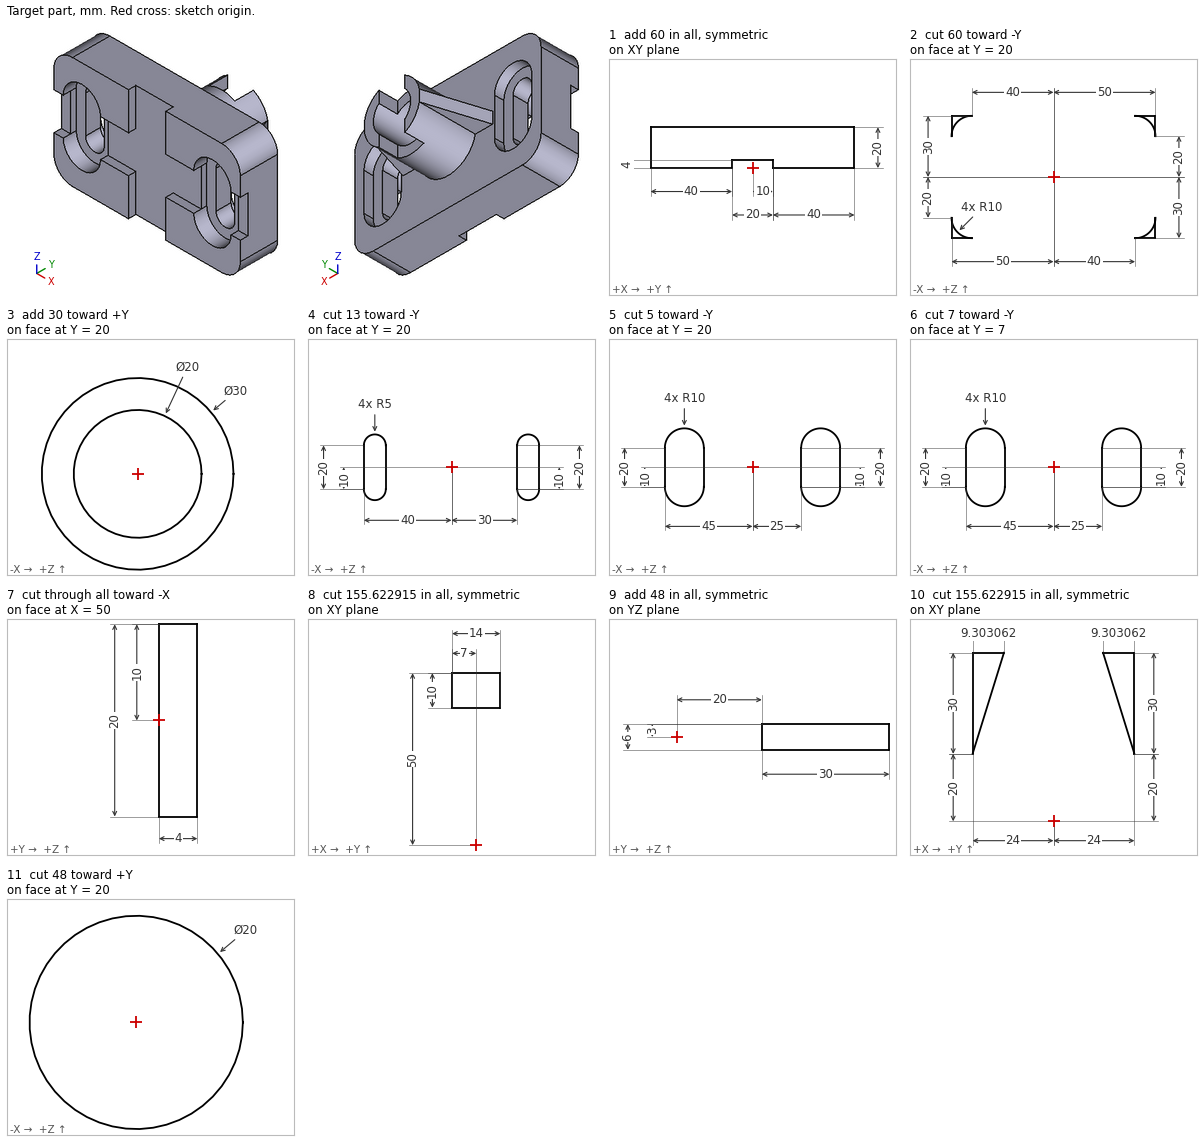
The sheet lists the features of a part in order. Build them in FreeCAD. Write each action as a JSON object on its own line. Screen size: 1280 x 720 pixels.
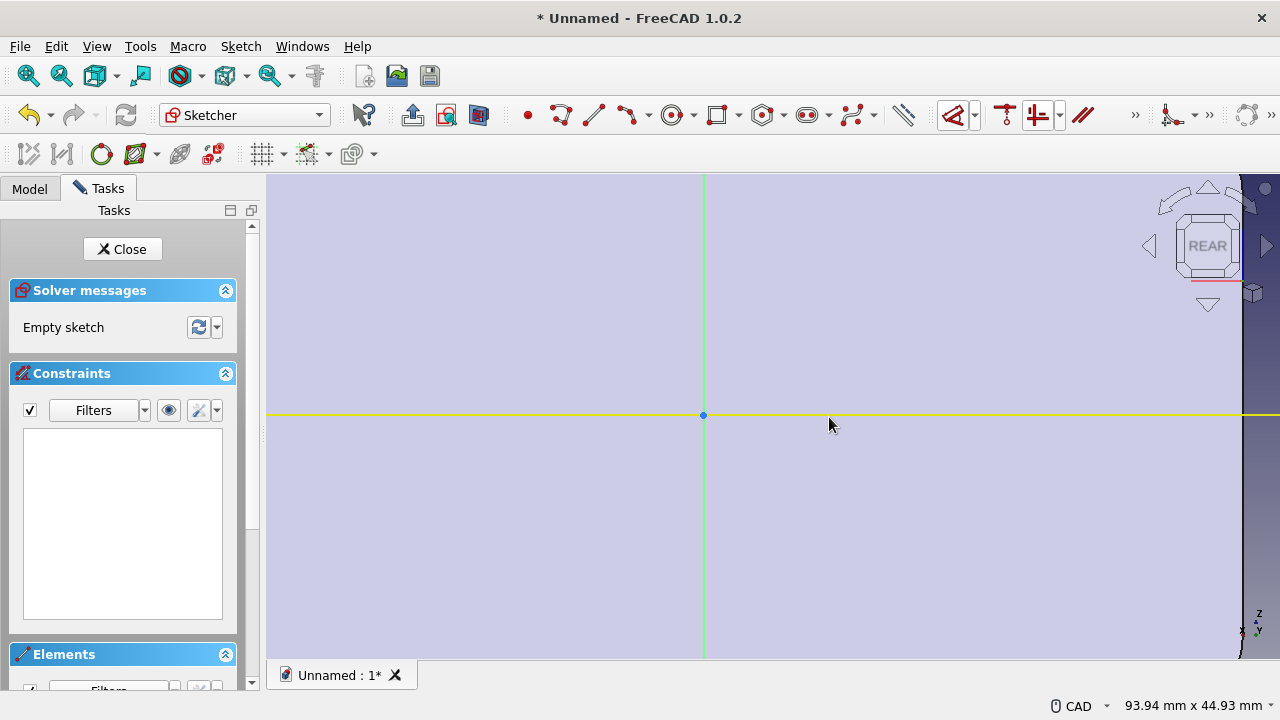
{"action": "key", "text": "g c"}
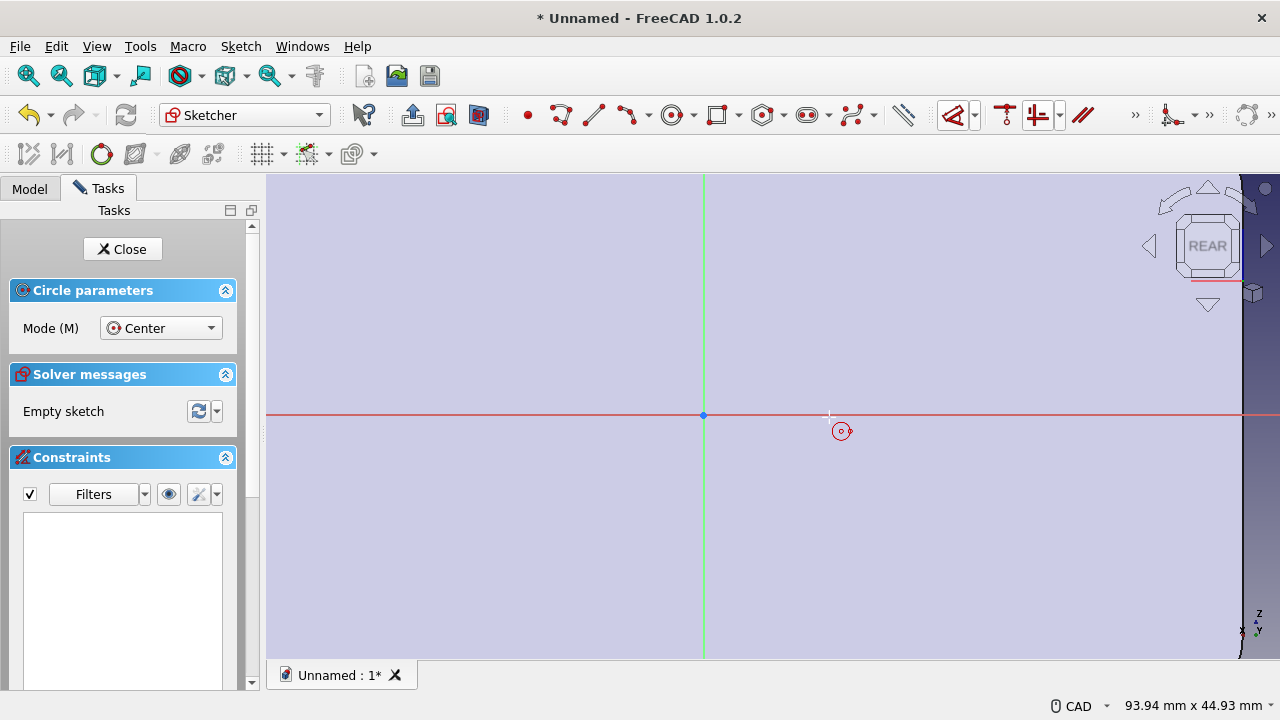
{"action": "left_click", "coordinate": [704, 415]}
{"action": "left_click", "coordinate": [818, 301]}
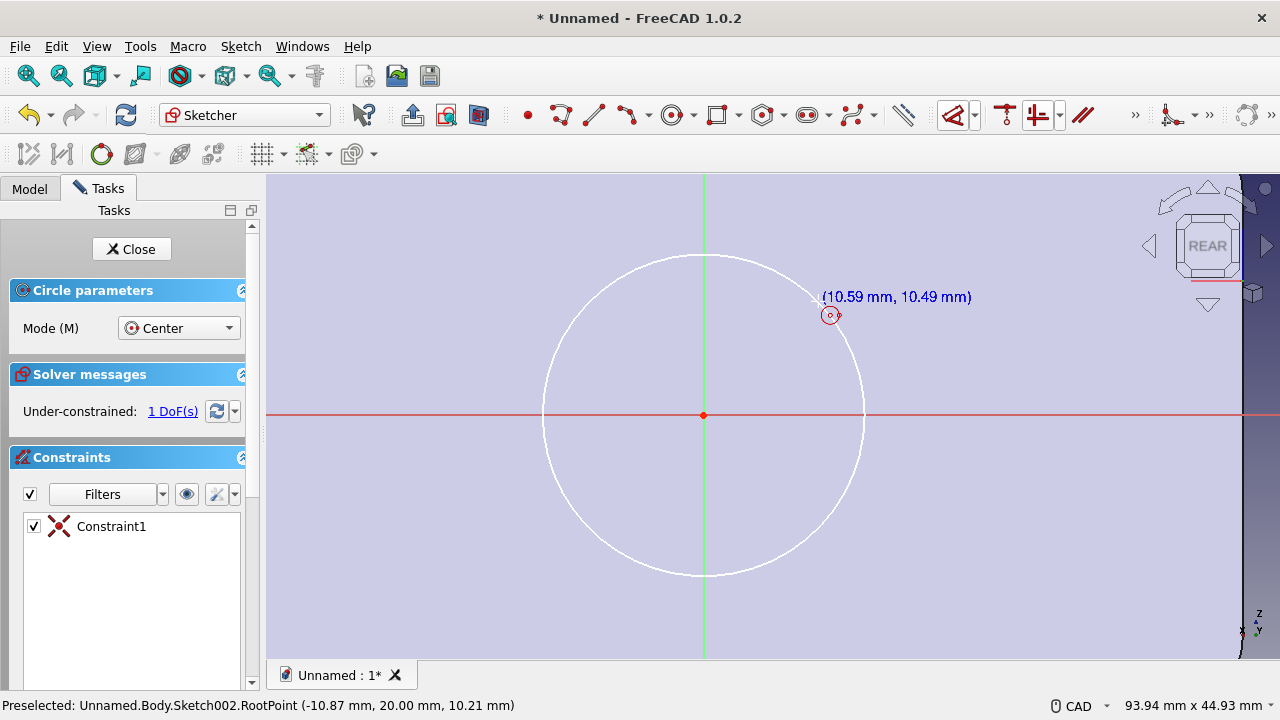
{"action": "left_click", "coordinate": [704, 415]}
{"action": "left_click", "coordinate": [780, 339]}
{"action": "key", "text": "Escape"}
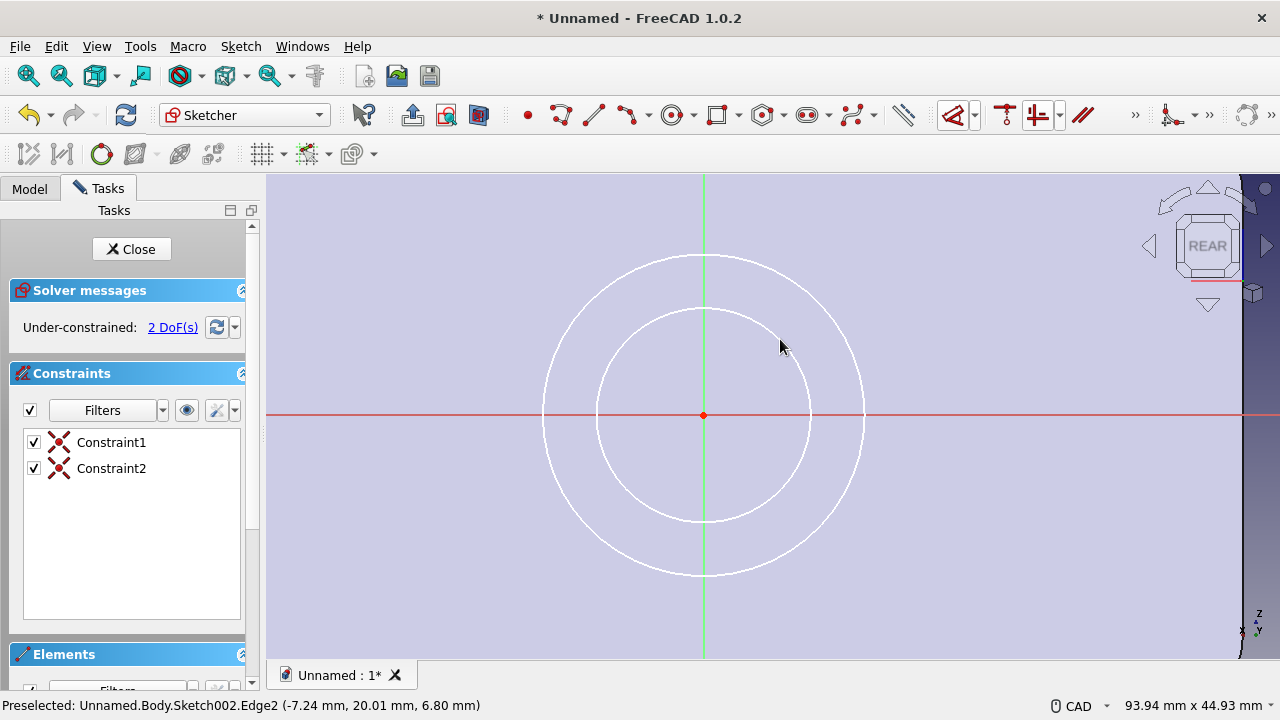
{"action": "left_click", "coordinate": [817, 301]}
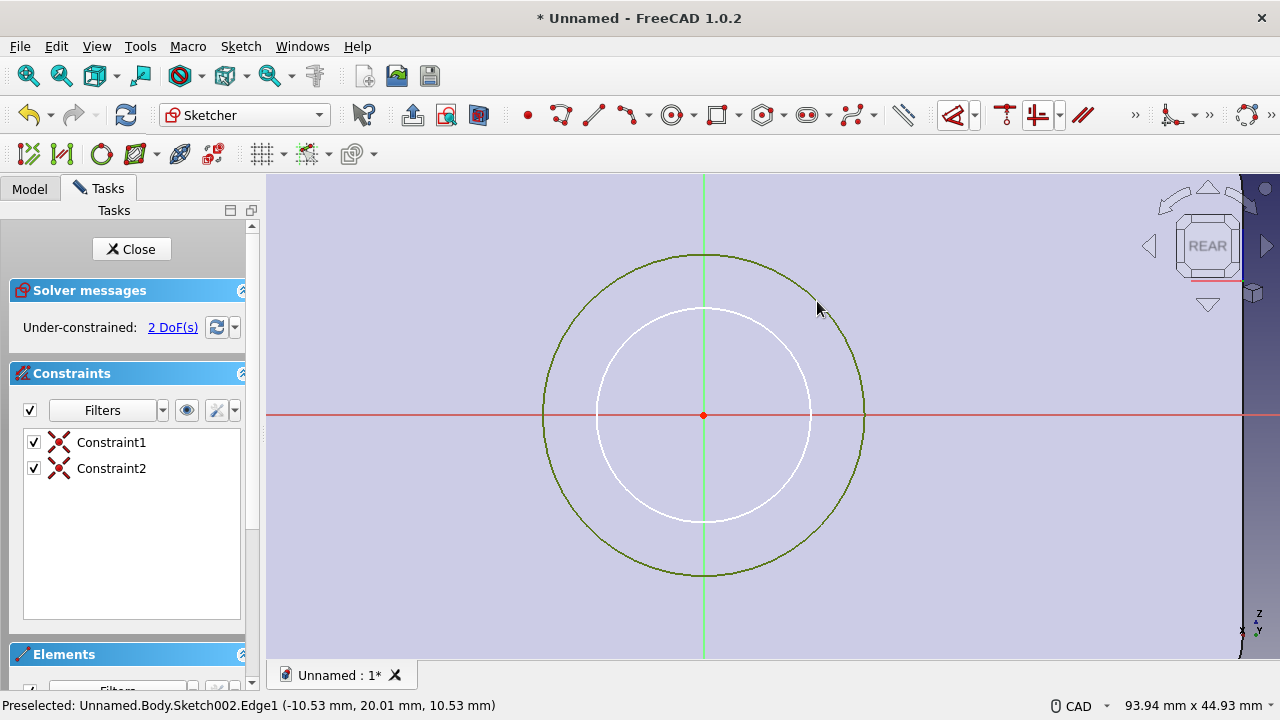
{"action": "key", "text": "k o"}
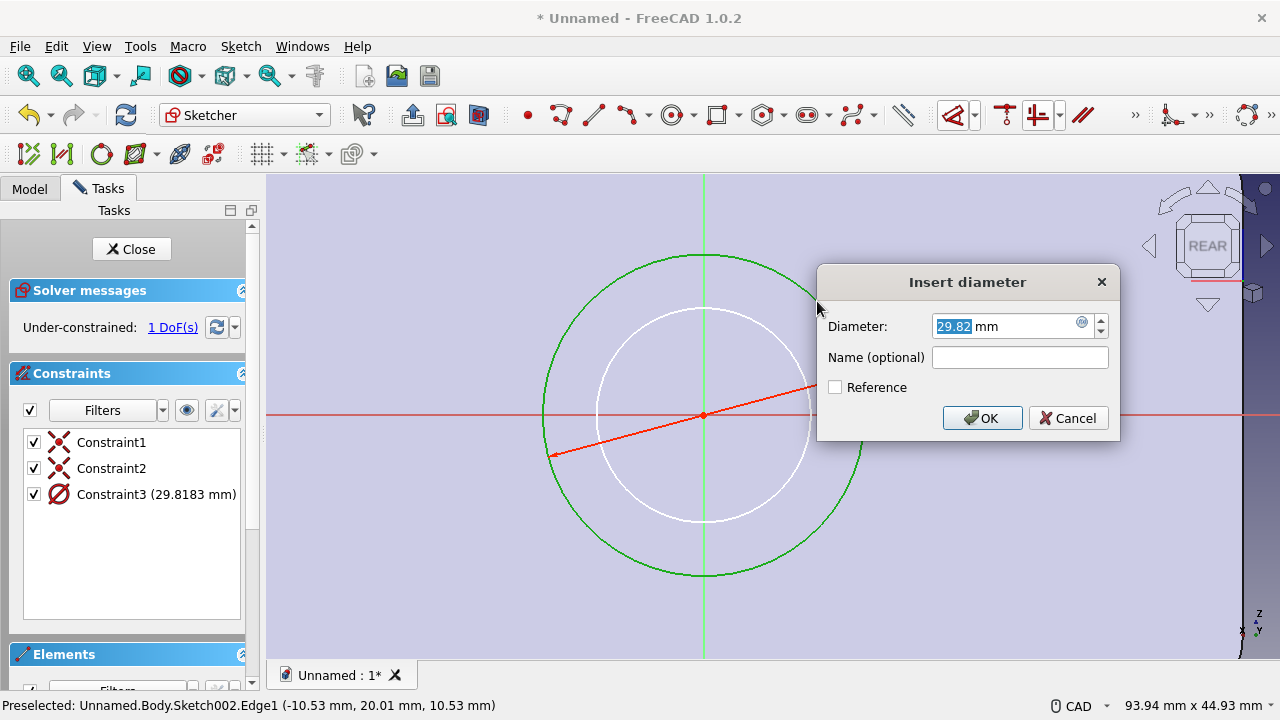
{"action": "type", "text": "30"}
{"action": "key", "text": "Return"}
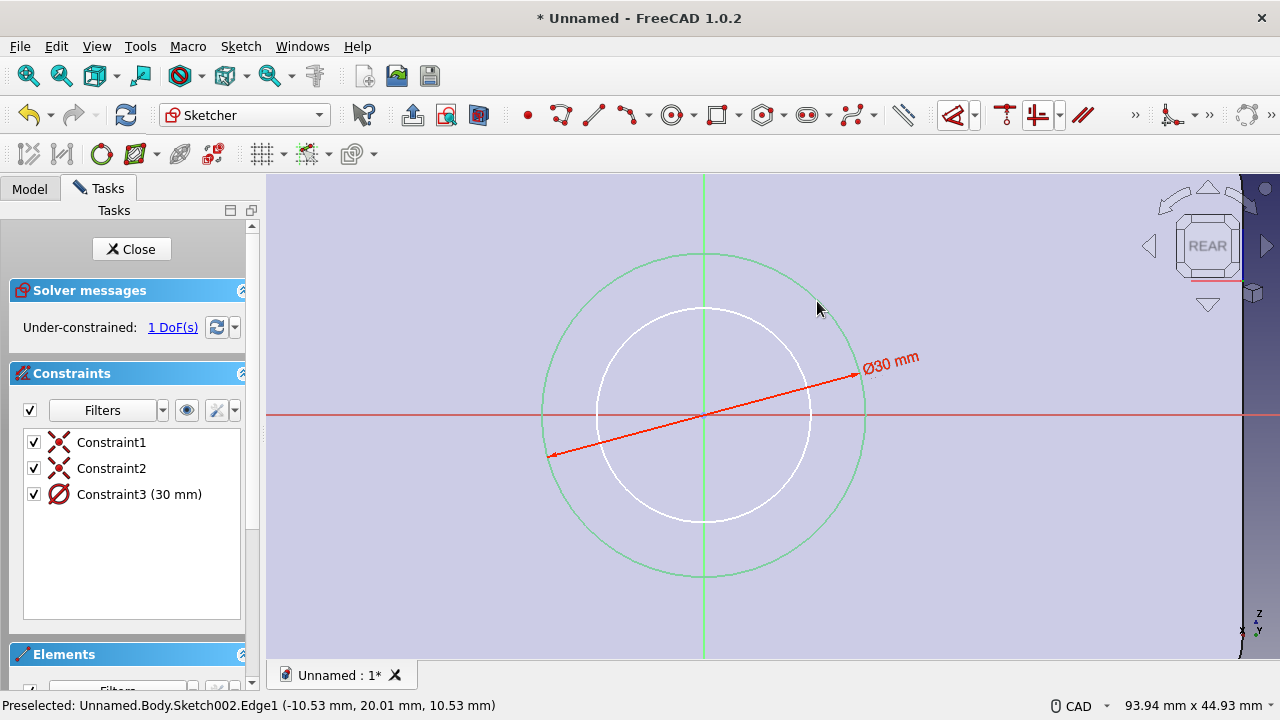
{"action": "left_click", "coordinate": [779, 339]}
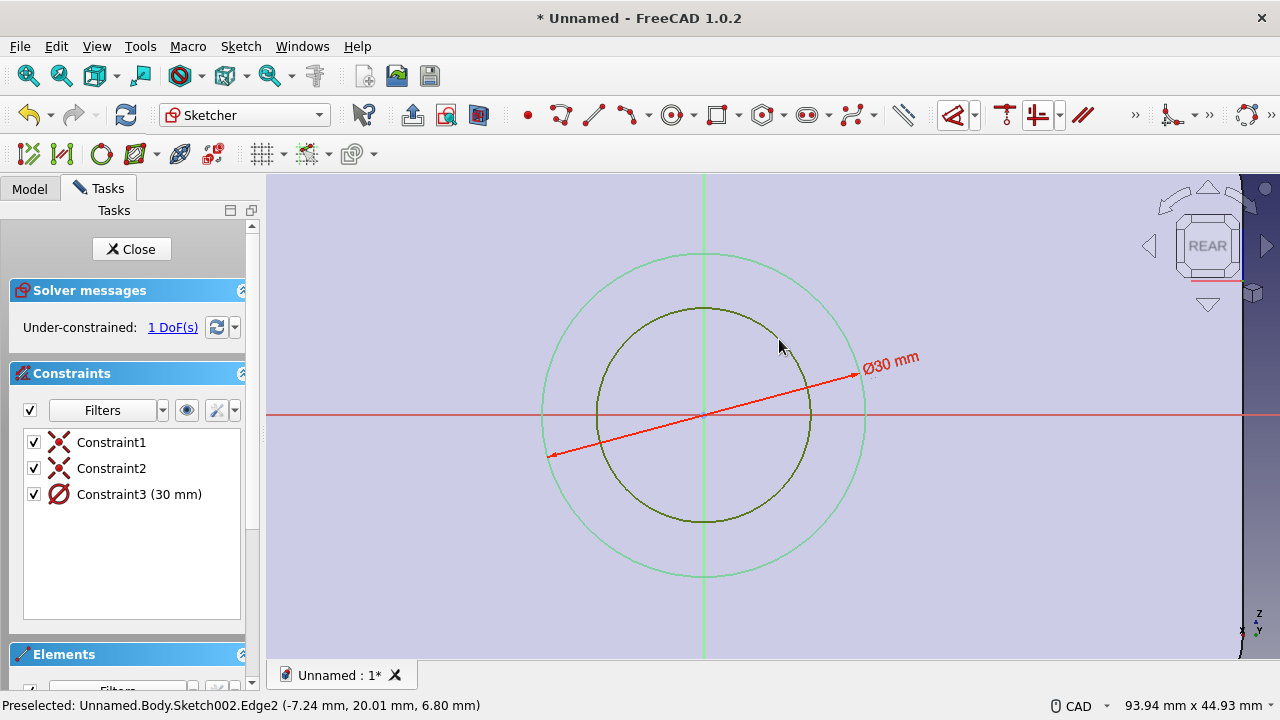
{"action": "key", "text": "k o"}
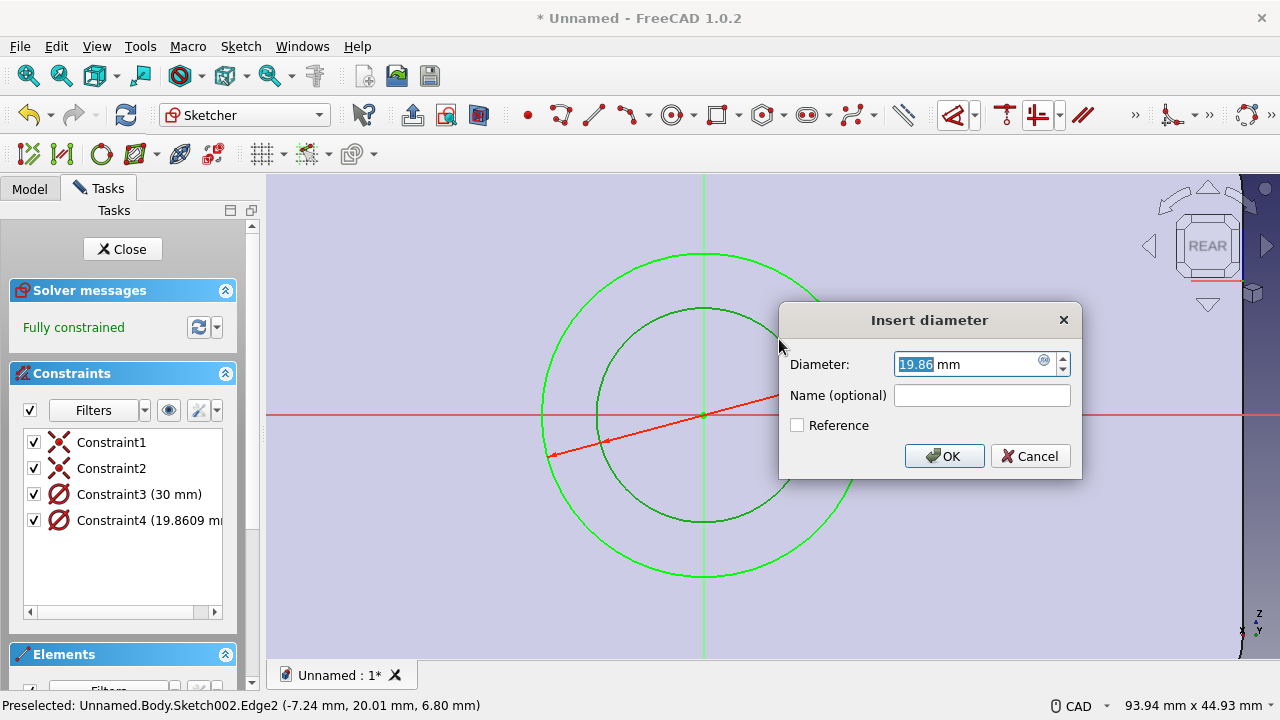
{"action": "type", "text": "20"}
{"action": "key", "text": "Return"}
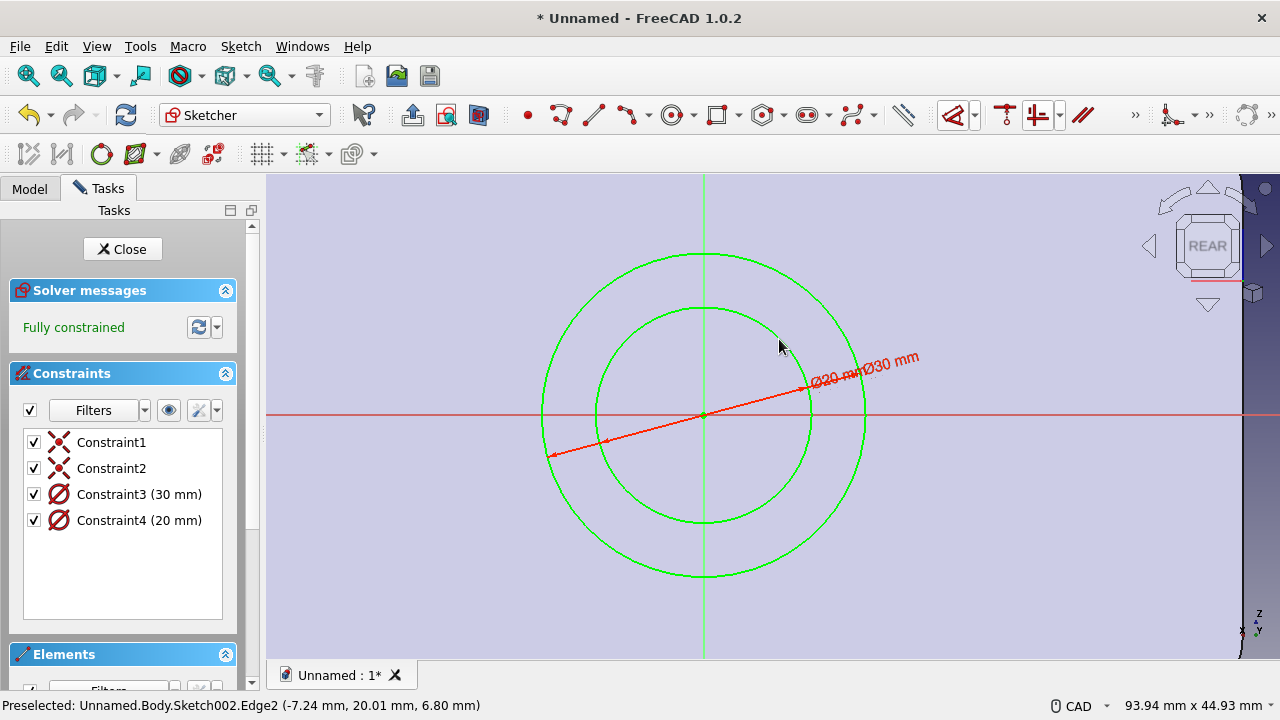
{"action": "left_click", "coordinate": [123, 249]}